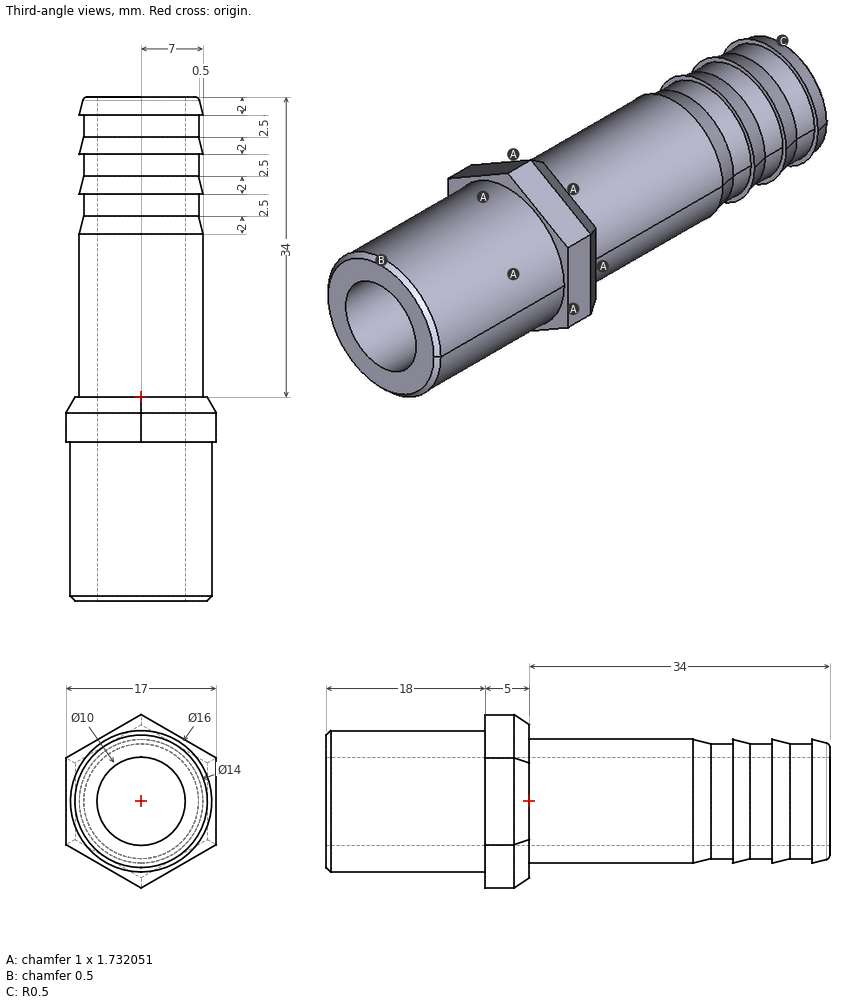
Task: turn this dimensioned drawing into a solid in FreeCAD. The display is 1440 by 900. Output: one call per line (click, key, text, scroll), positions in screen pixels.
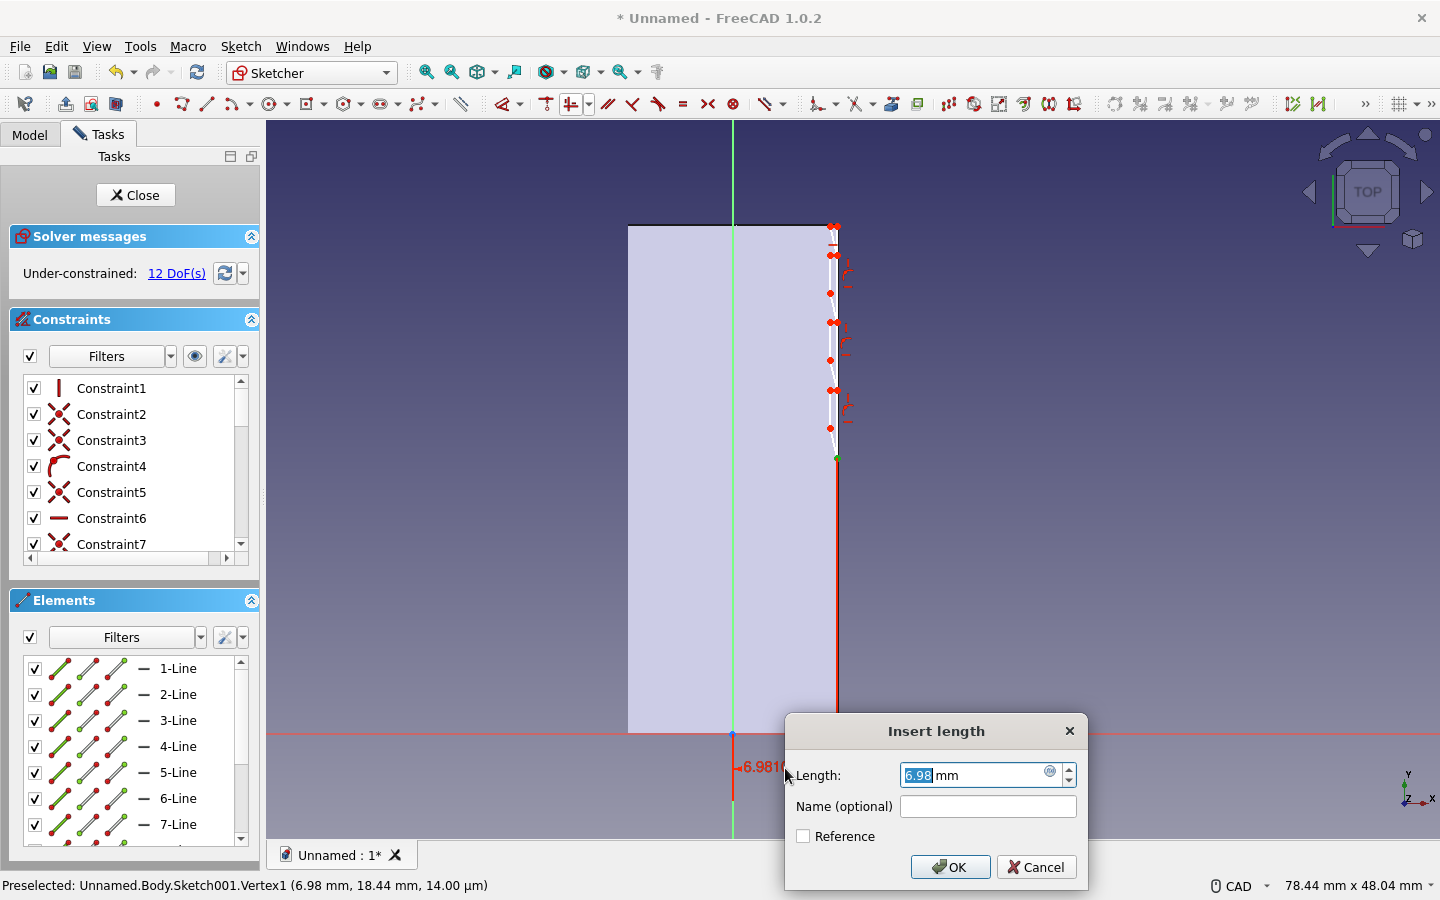
text(7)
key(Return)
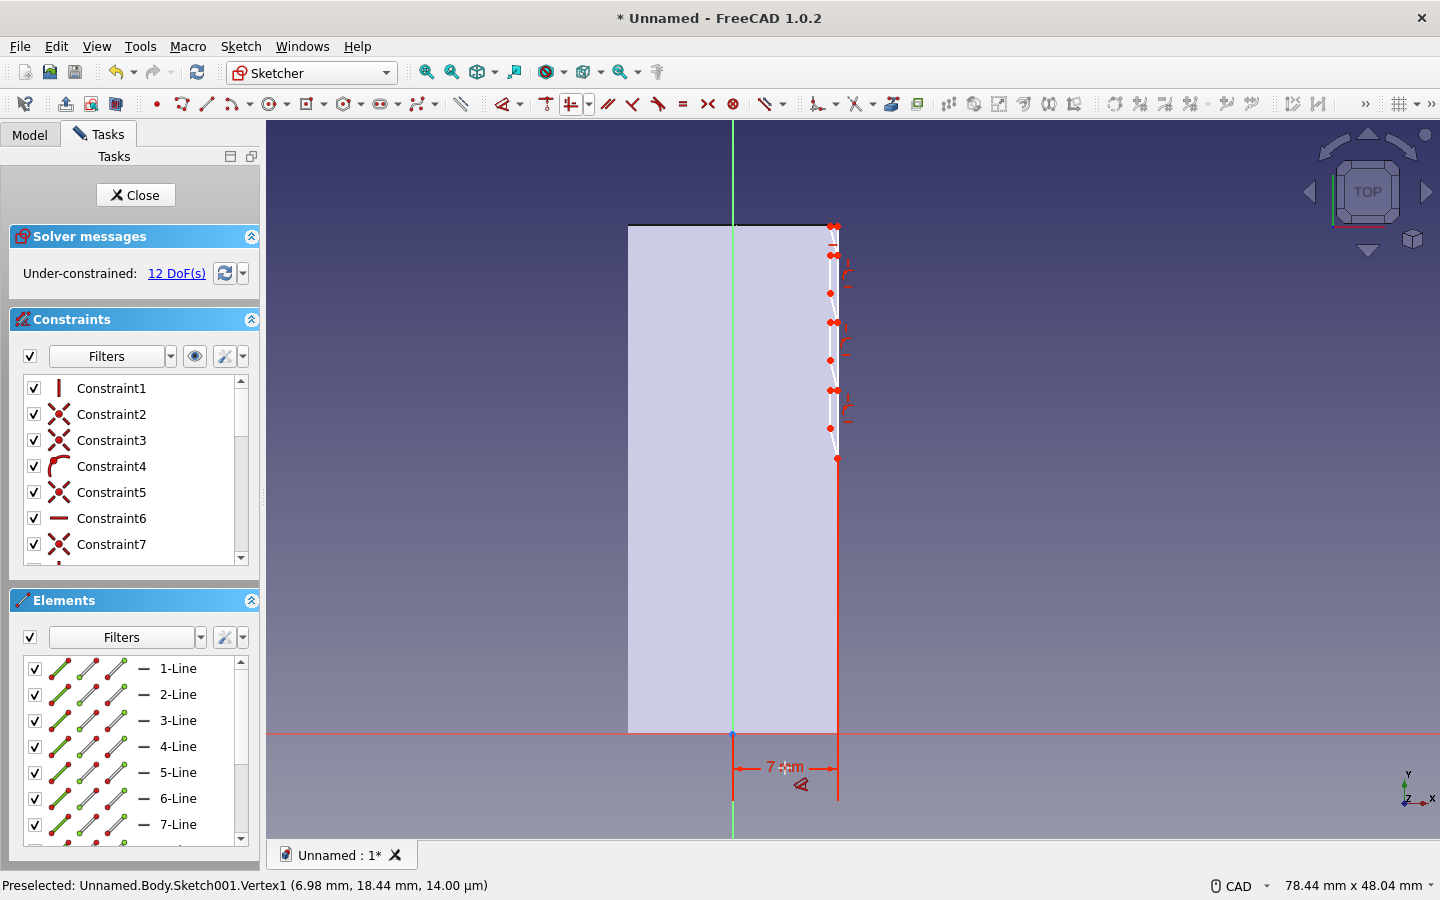
scroll(832, 232, up, 5)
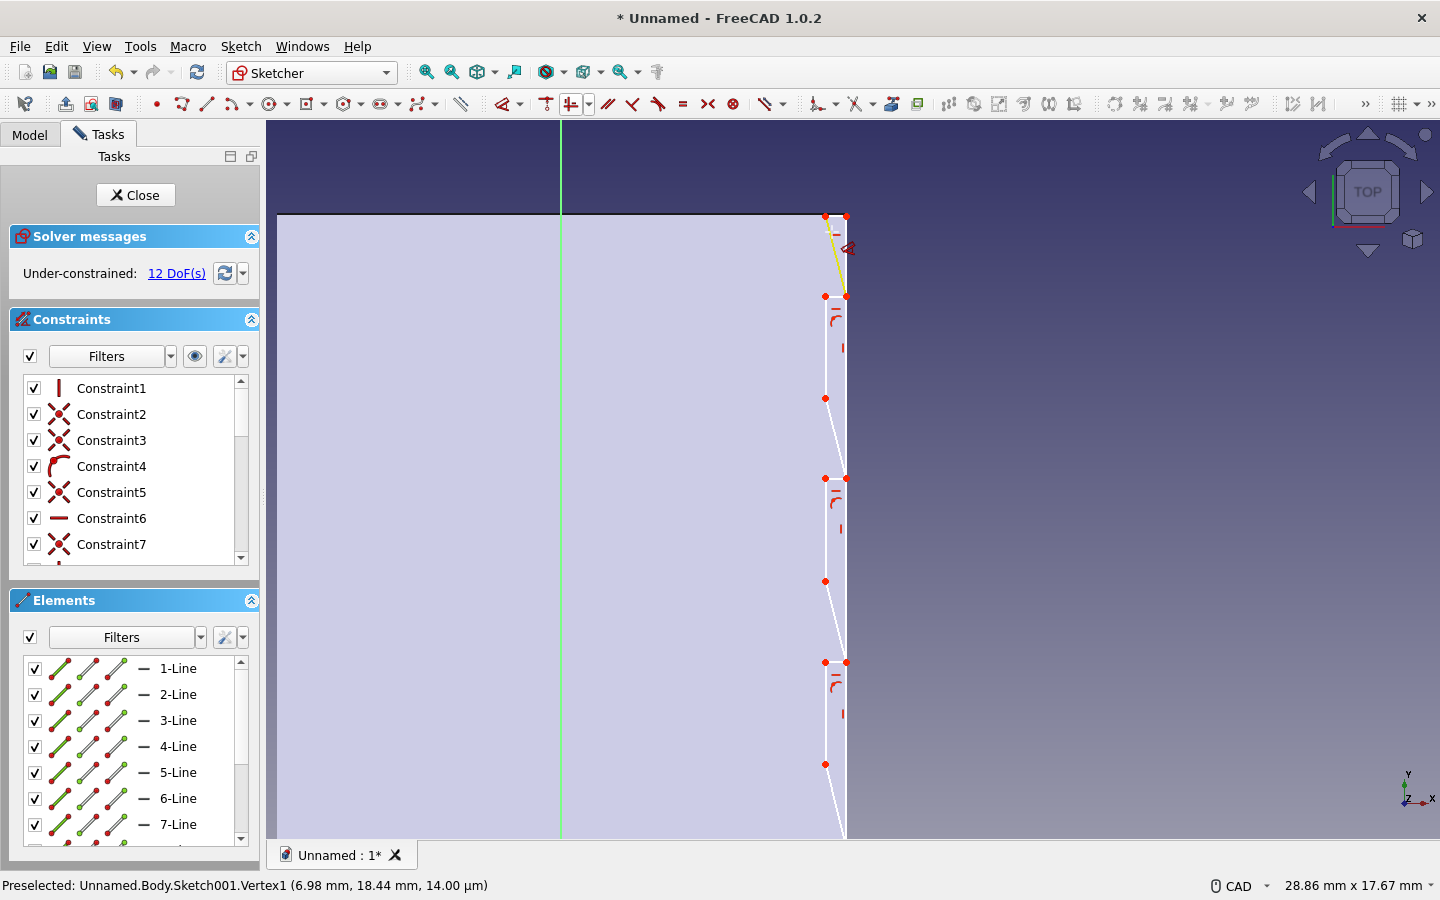
click(830, 232)
click(880, 257)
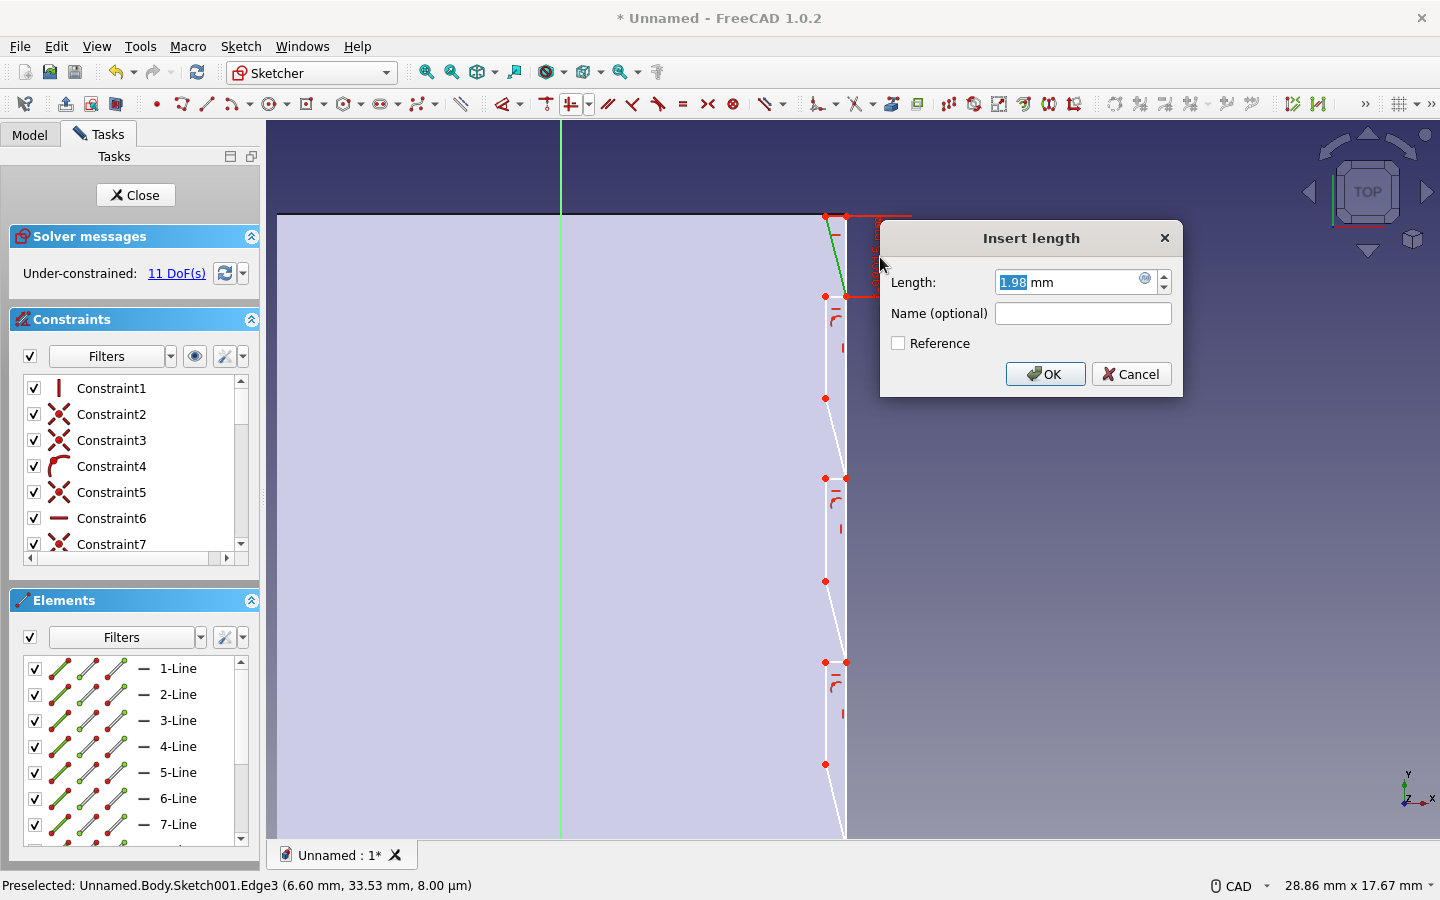
text(2)
key(Return)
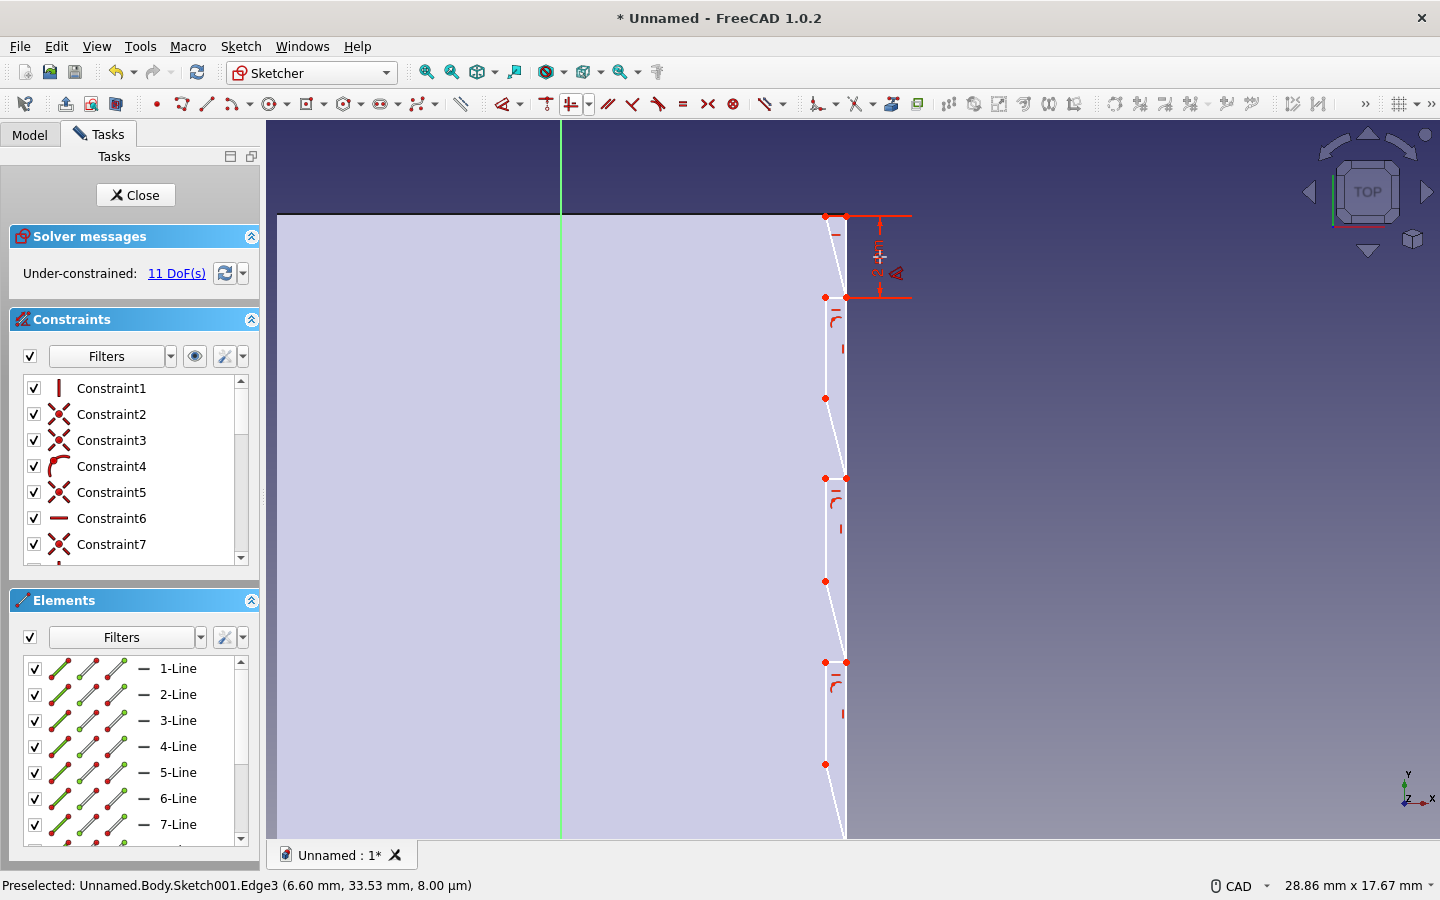
click(832, 422)
click(880, 439)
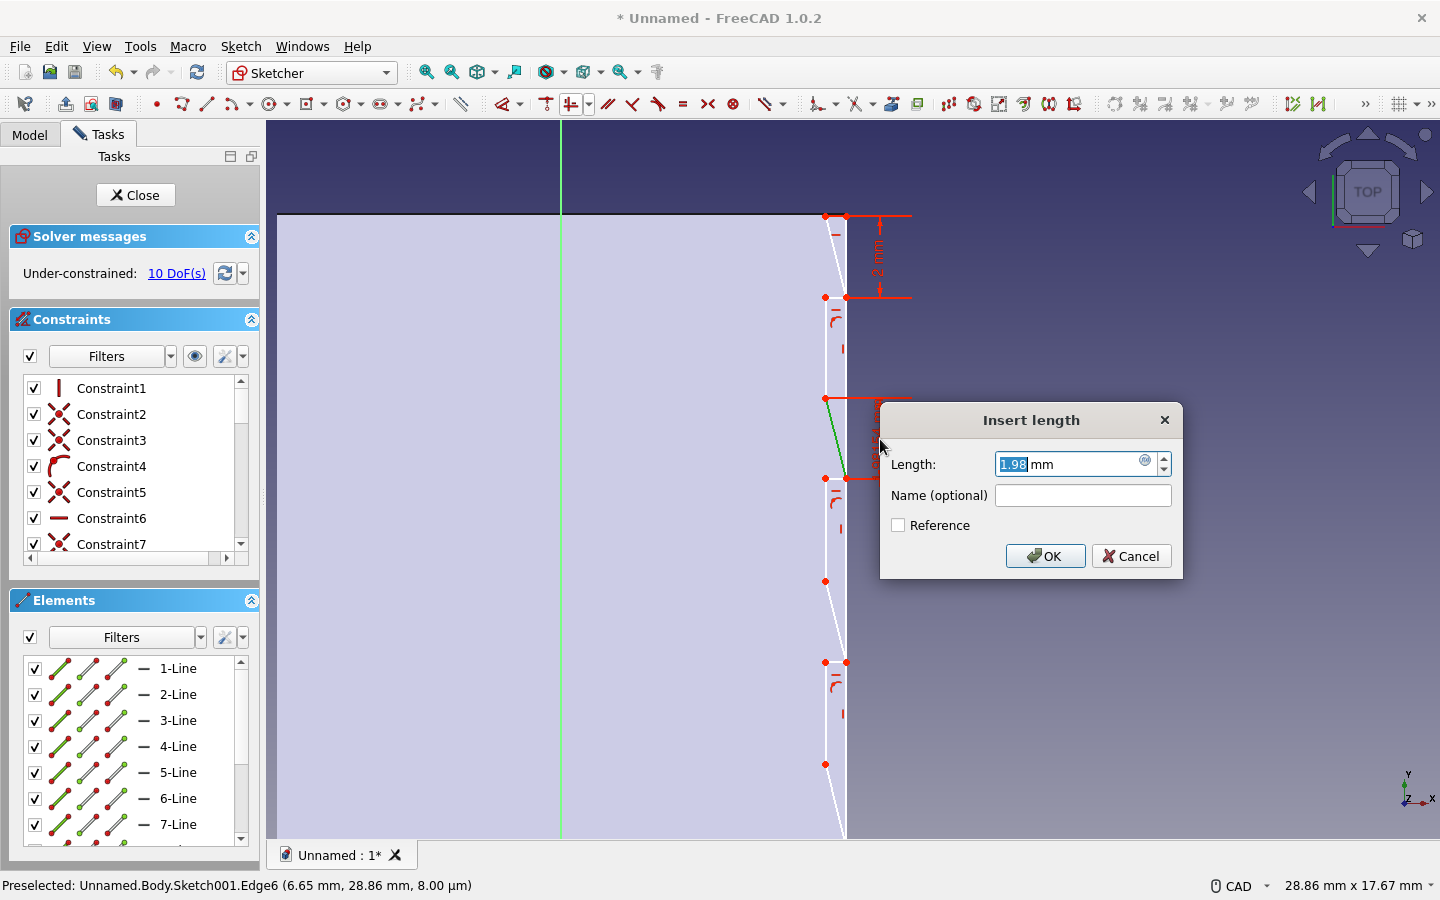
text(2)
key(Return)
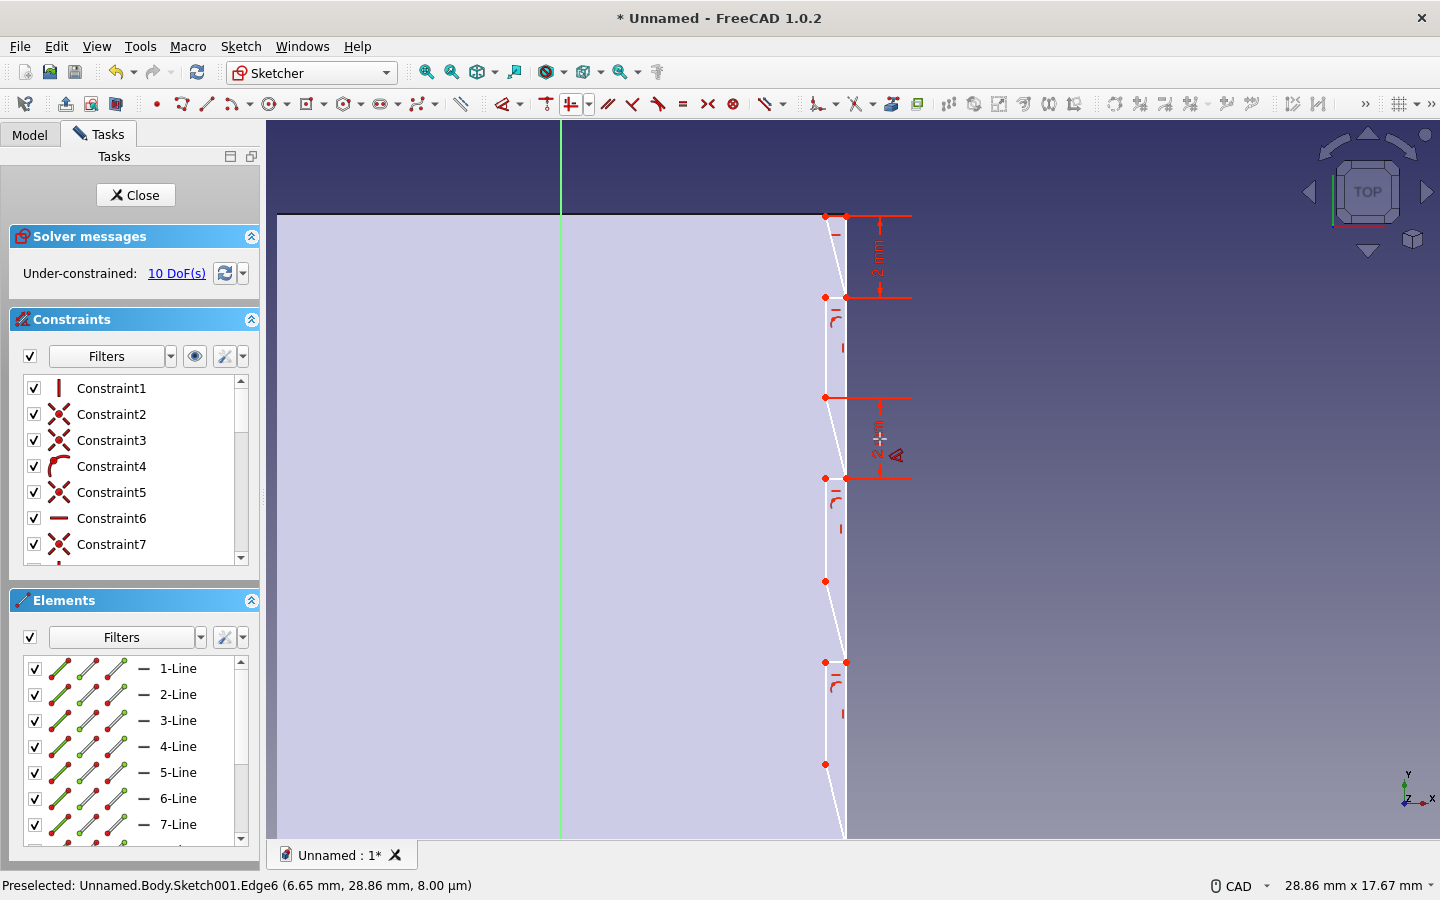
click(832, 606)
click(880, 622)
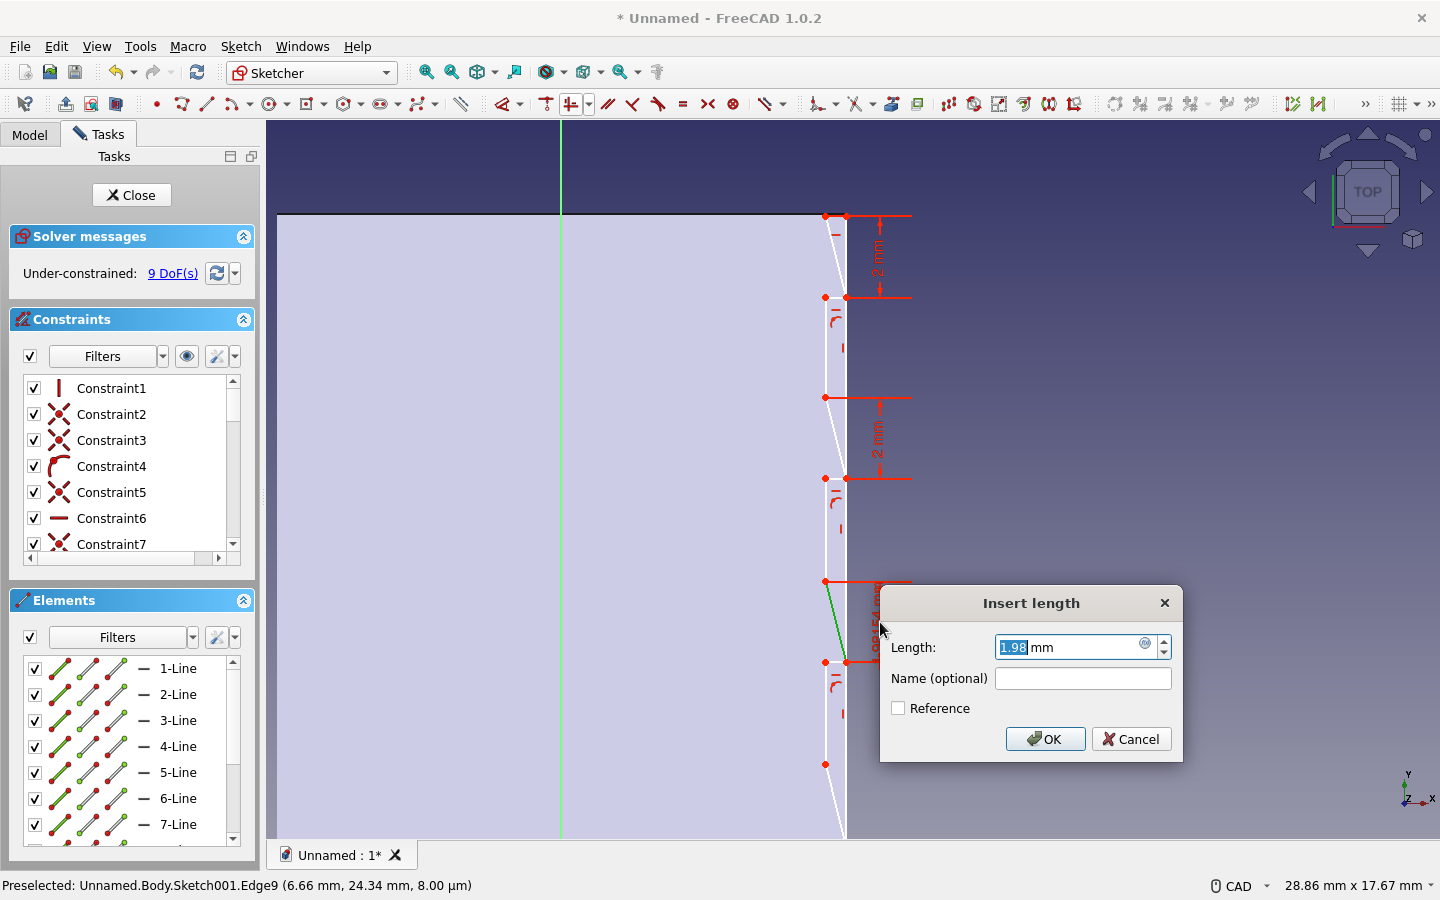
text(2)
key(Return)